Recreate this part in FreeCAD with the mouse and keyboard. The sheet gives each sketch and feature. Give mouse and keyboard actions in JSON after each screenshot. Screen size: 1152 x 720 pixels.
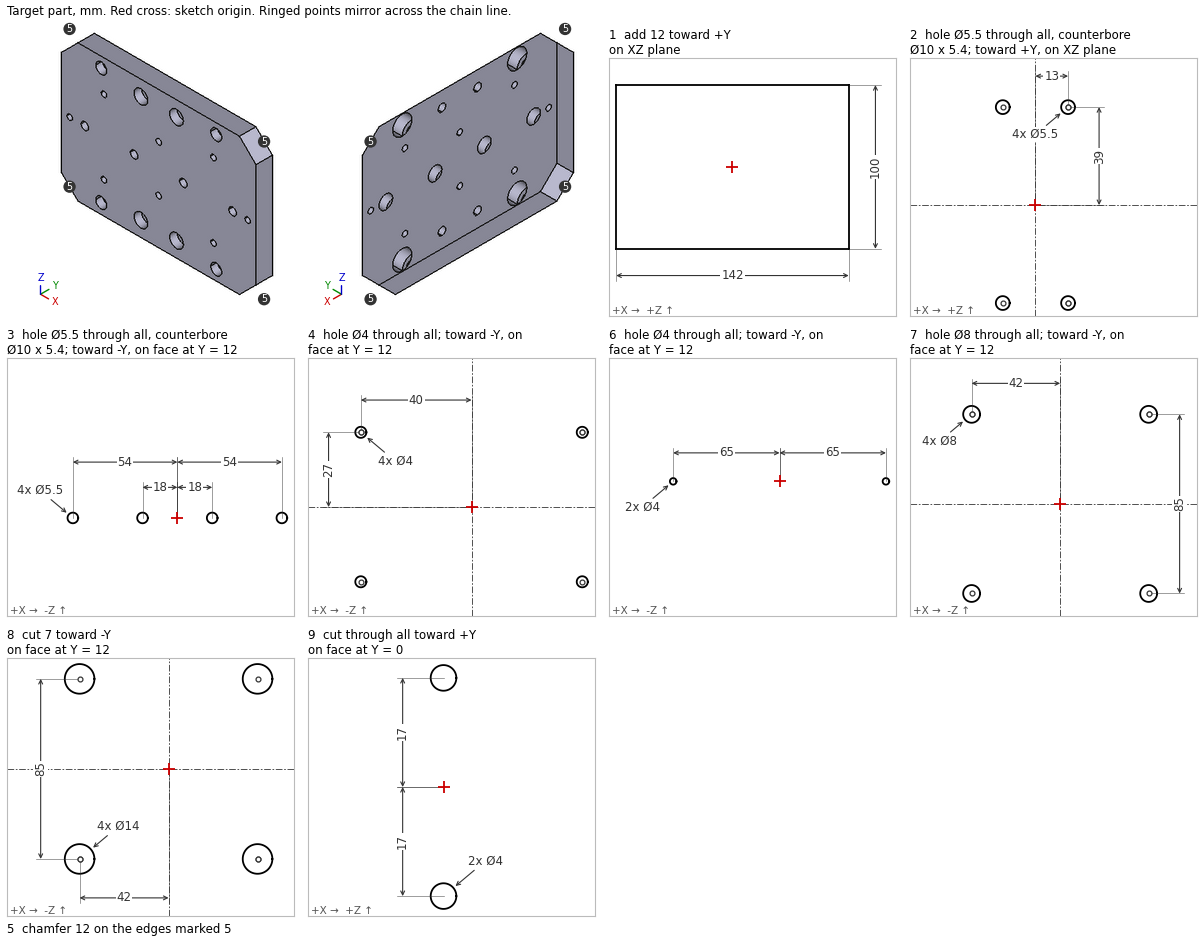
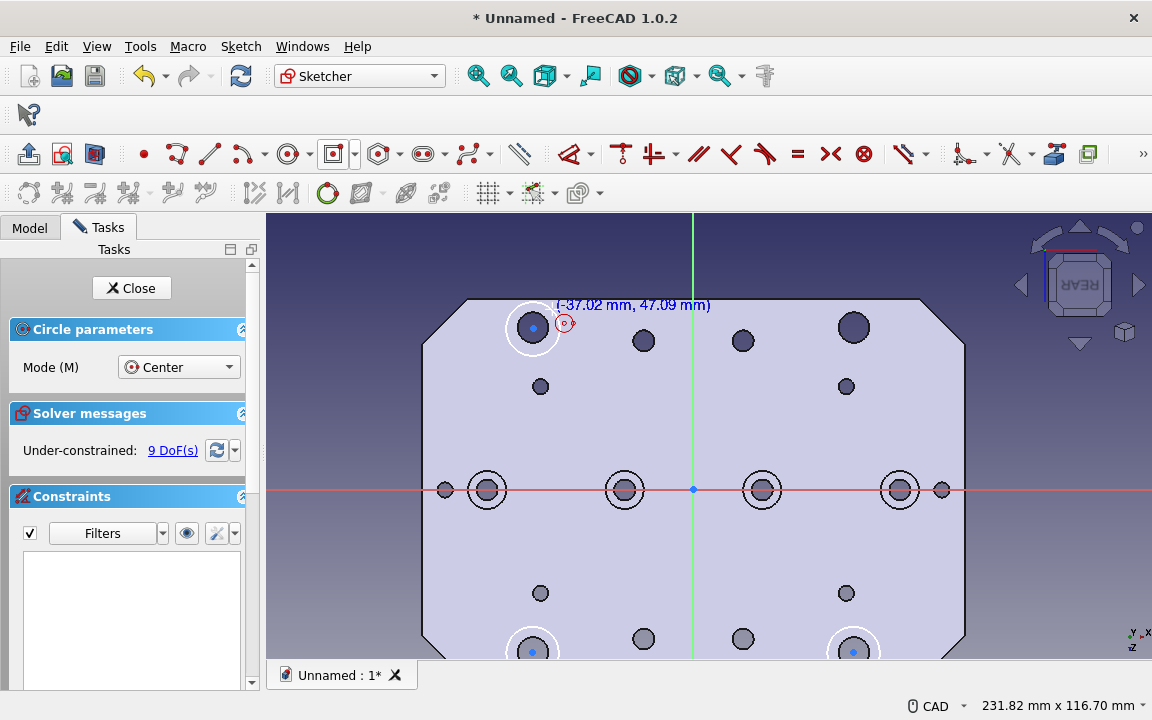
{"action": "left_click", "coordinate": [854, 328]}
{"action": "left_click", "coordinate": [873, 309]}
{"action": "key", "text": "Escape"}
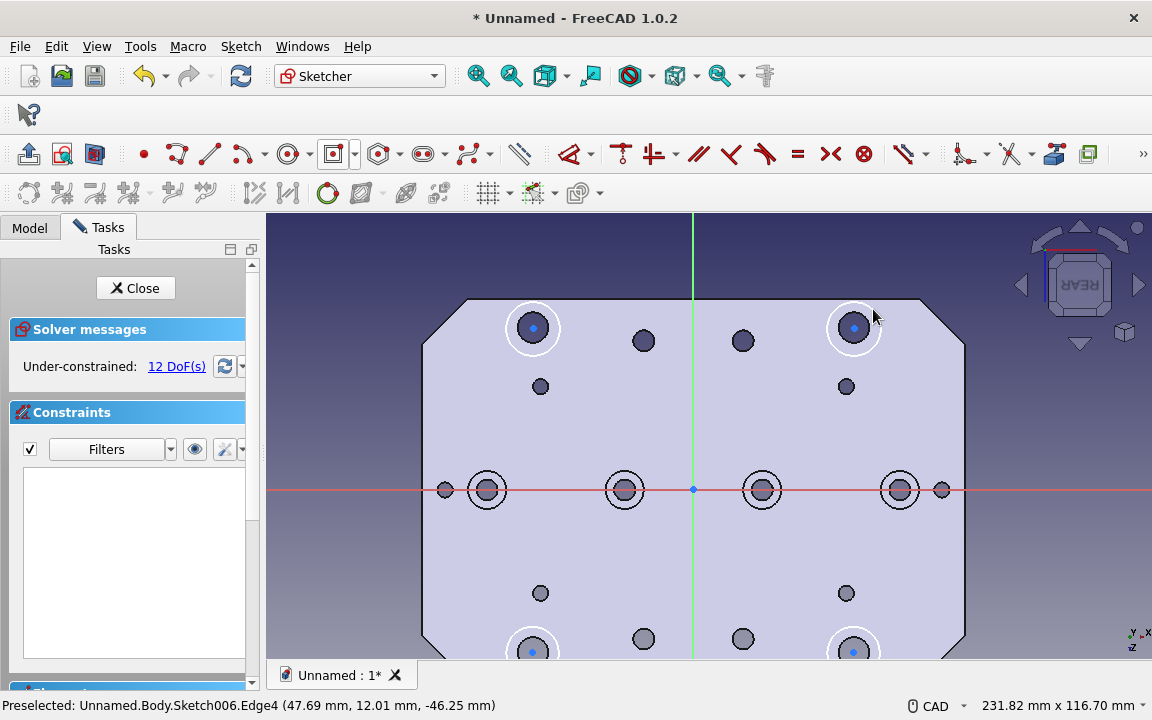
{"action": "left_click", "coordinate": [533, 627]}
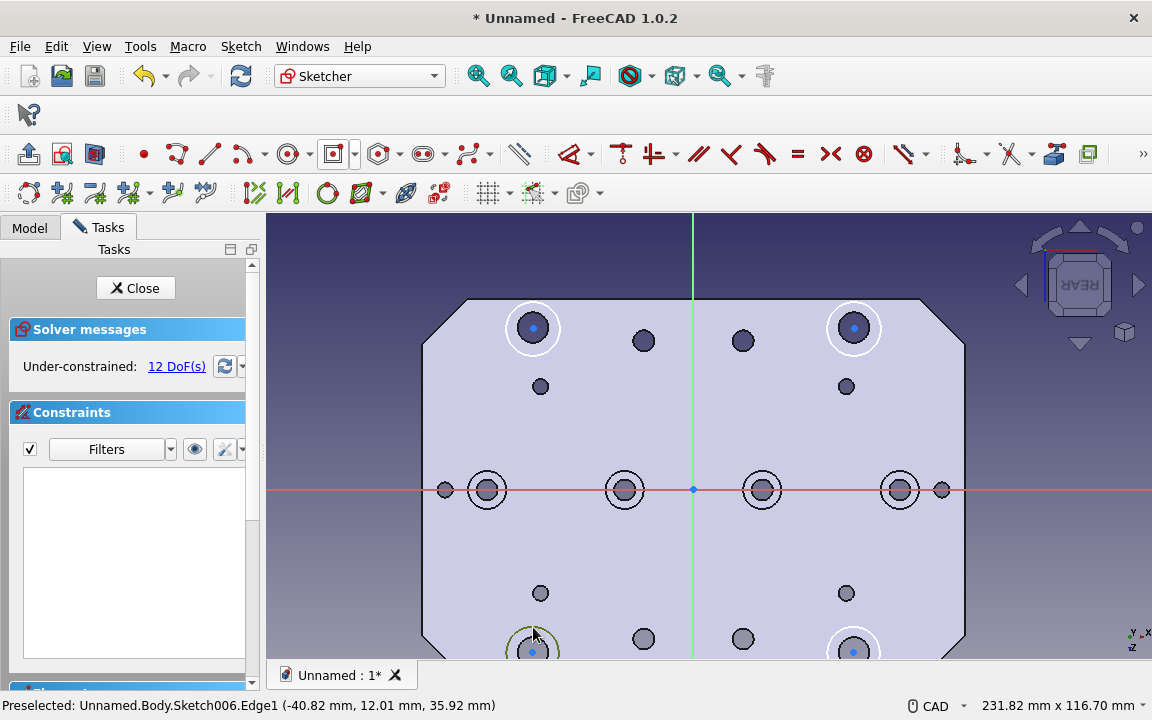
{"action": "left_click", "coordinate": [854, 627]}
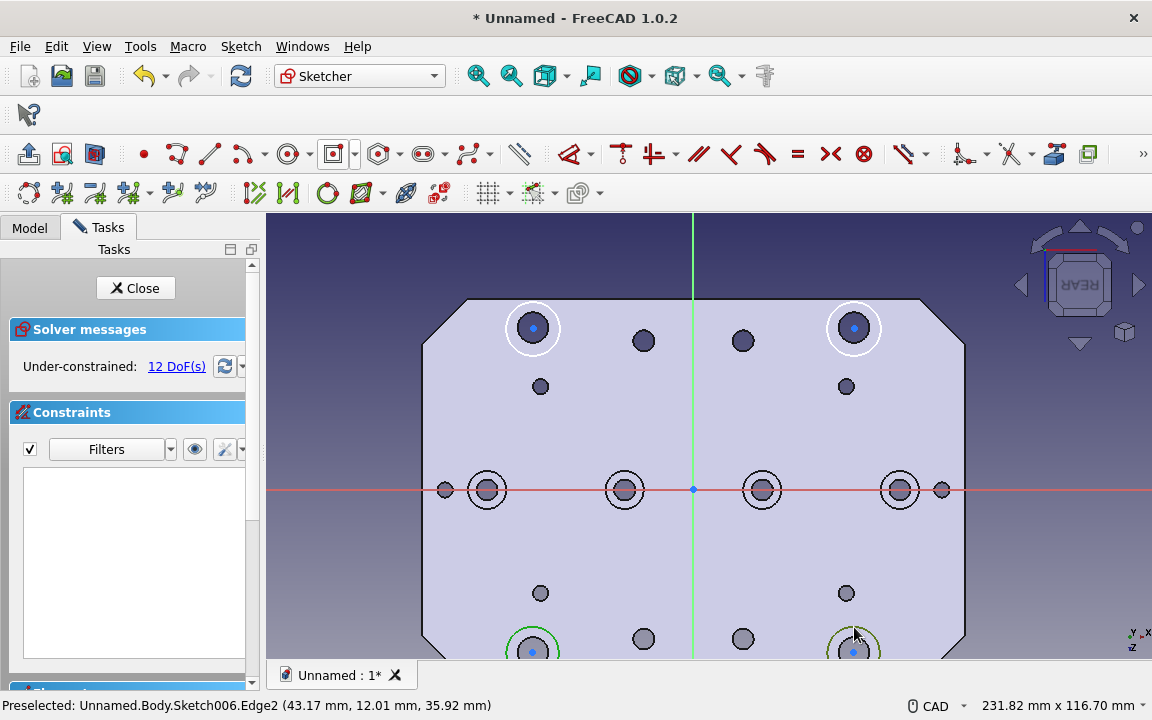
{"action": "left_click", "coordinate": [552, 310]}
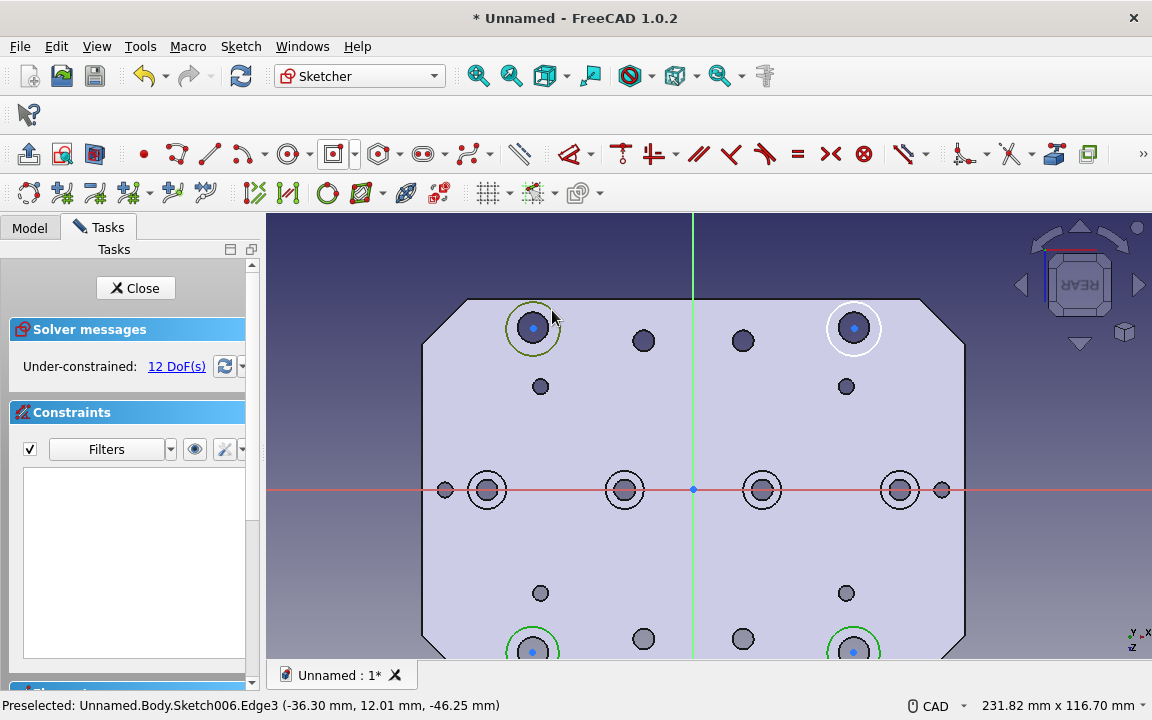
{"action": "left_click", "coordinate": [873, 310]}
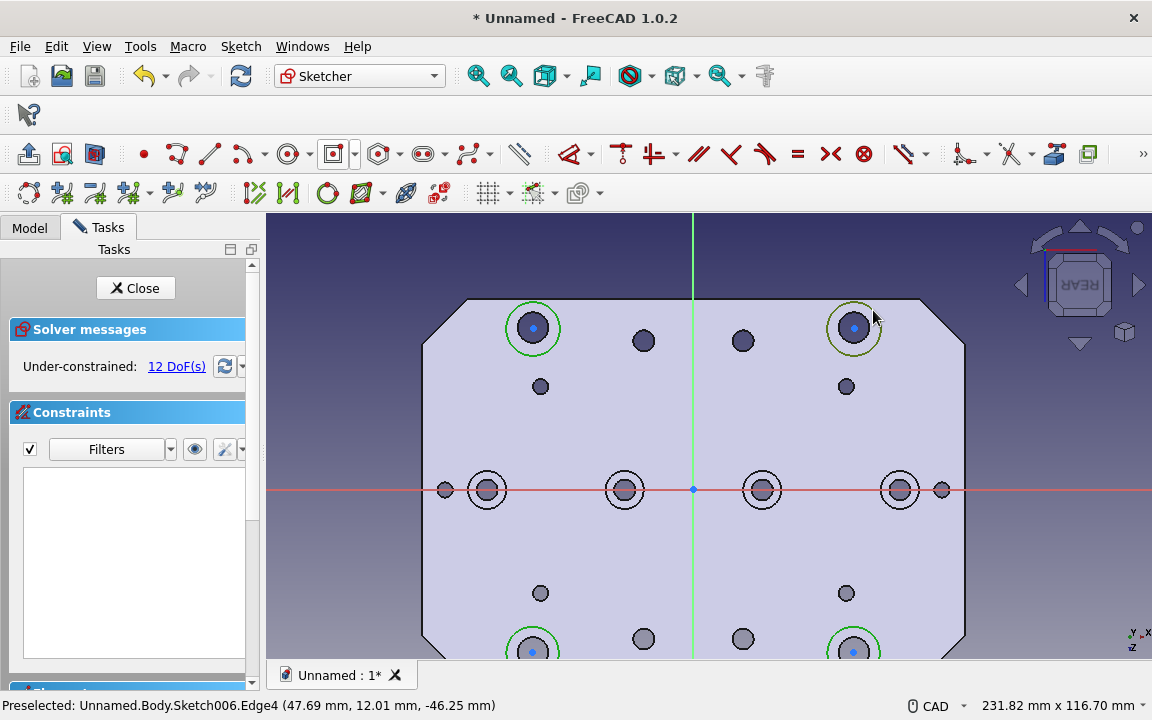
{"action": "left_click", "coordinate": [798, 154]}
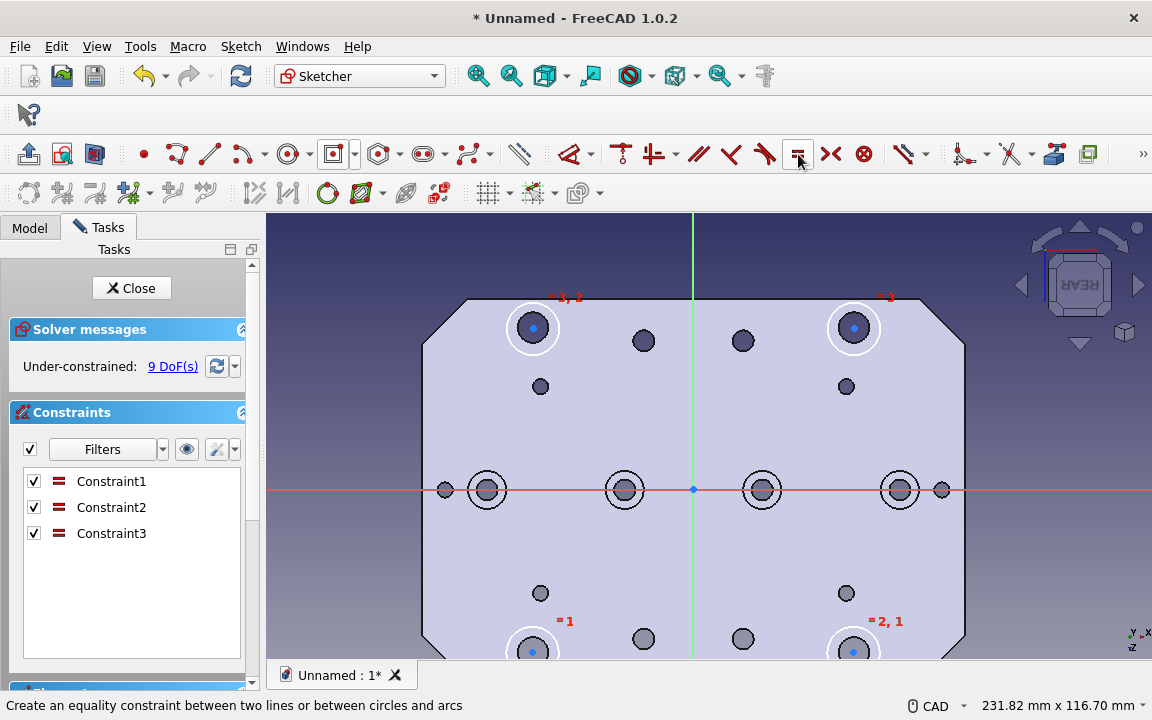
{"action": "scroll", "coordinate": [533, 326], "scroll_direction": "down", "scroll_amount": 2}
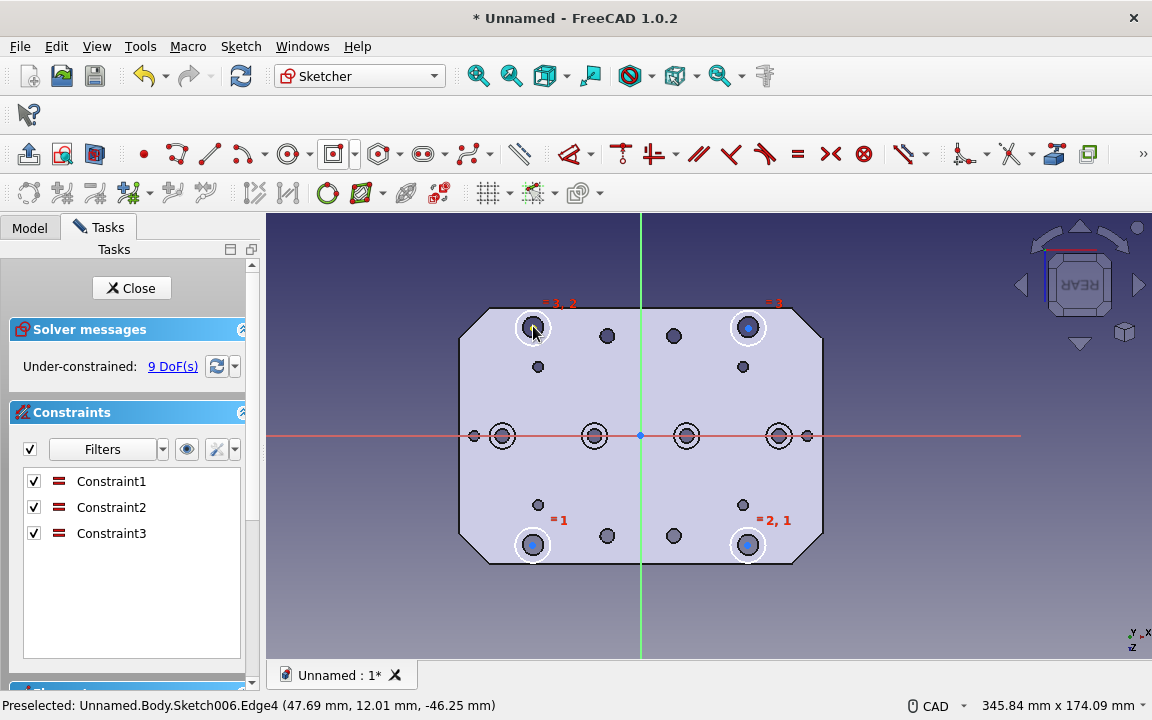
{"action": "left_click", "coordinate": [533, 545]}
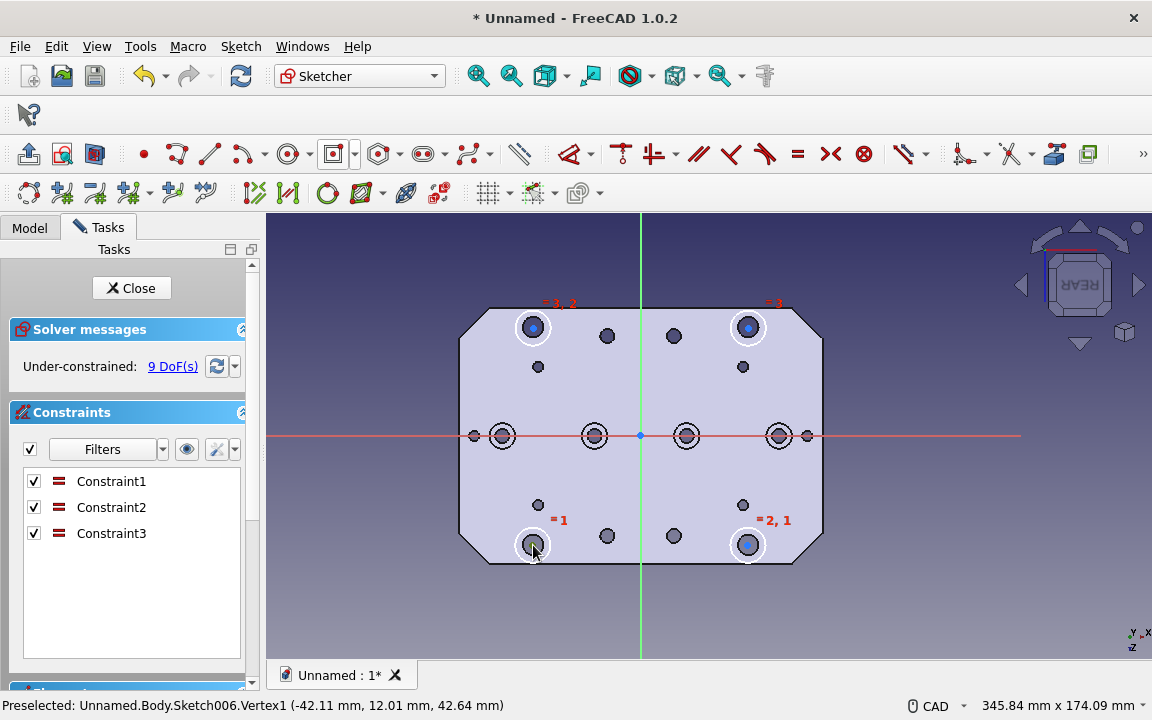
{"action": "left_click", "coordinate": [748, 545]}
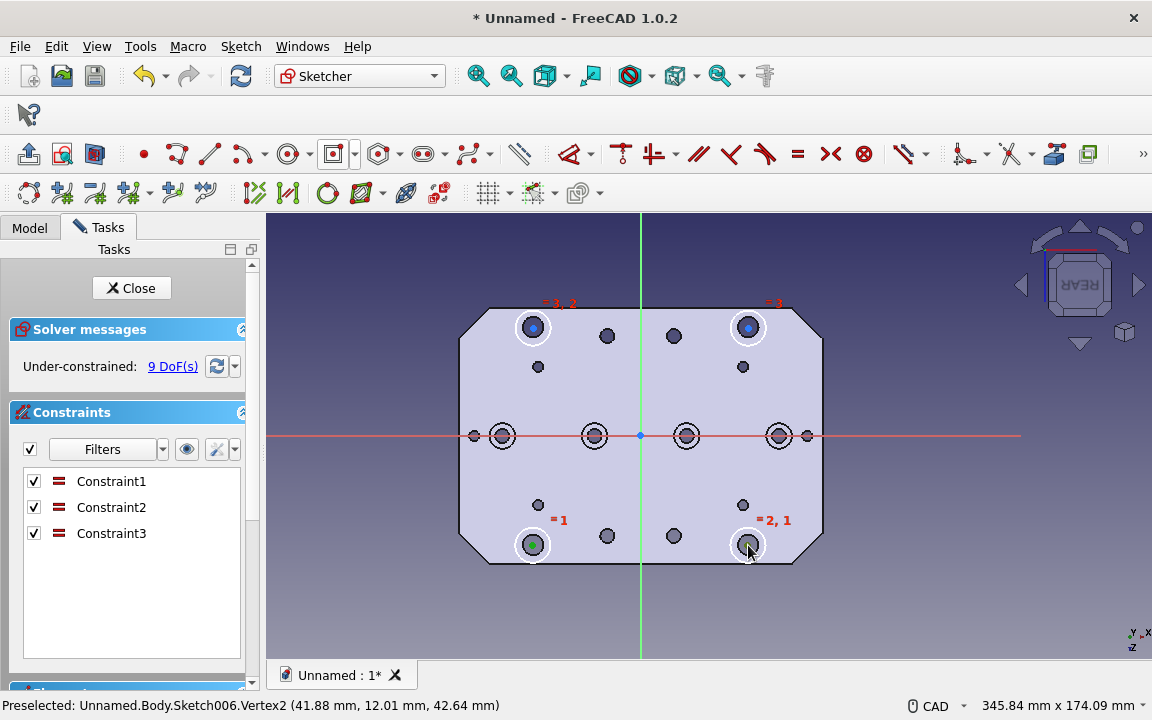
{"action": "left_click", "coordinate": [641, 603]}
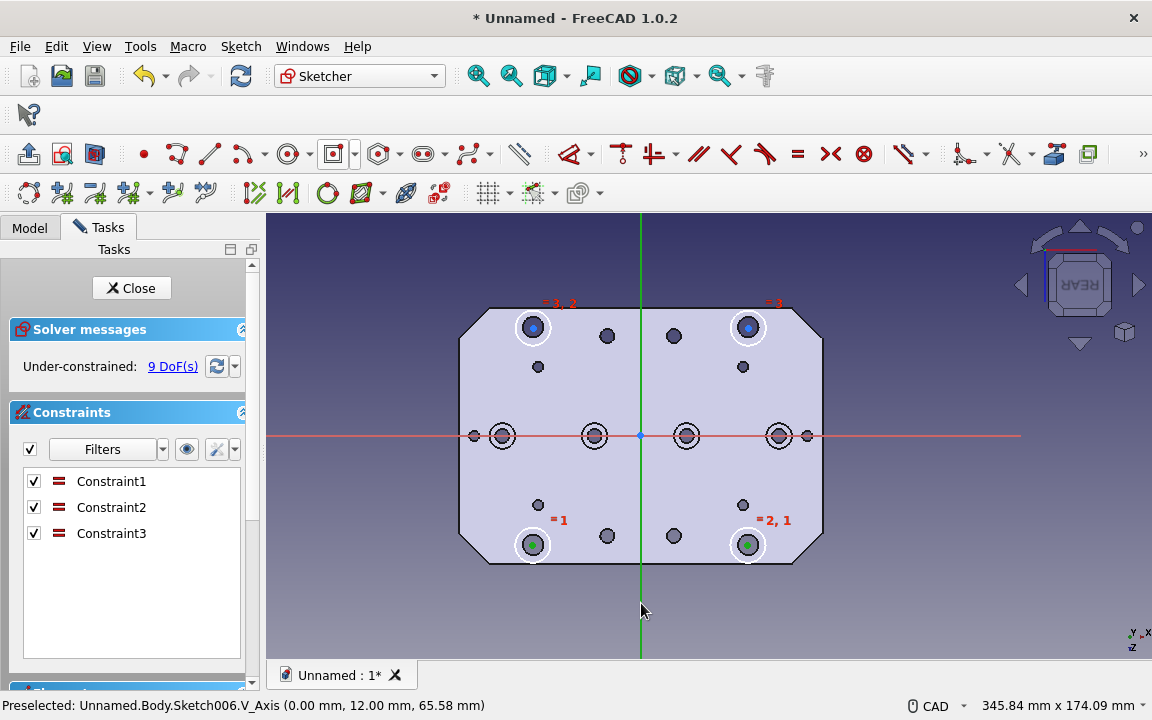
{"action": "left_click", "coordinate": [831, 154]}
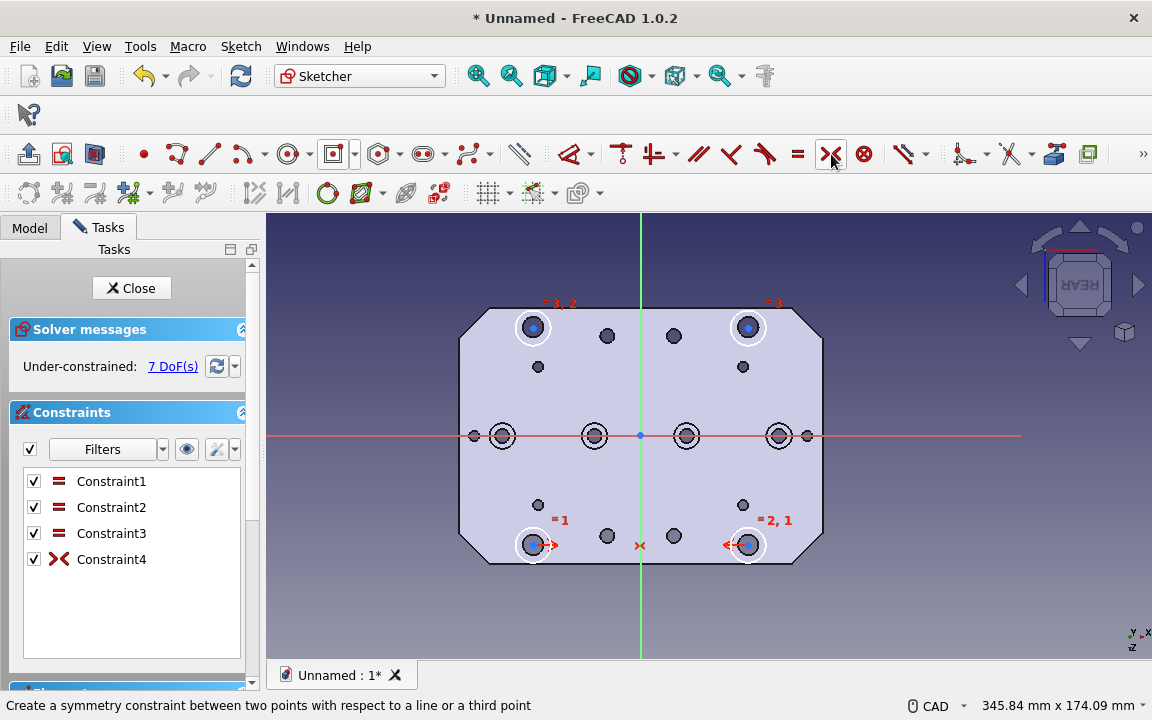
{"action": "left_click", "coordinate": [533, 545]}